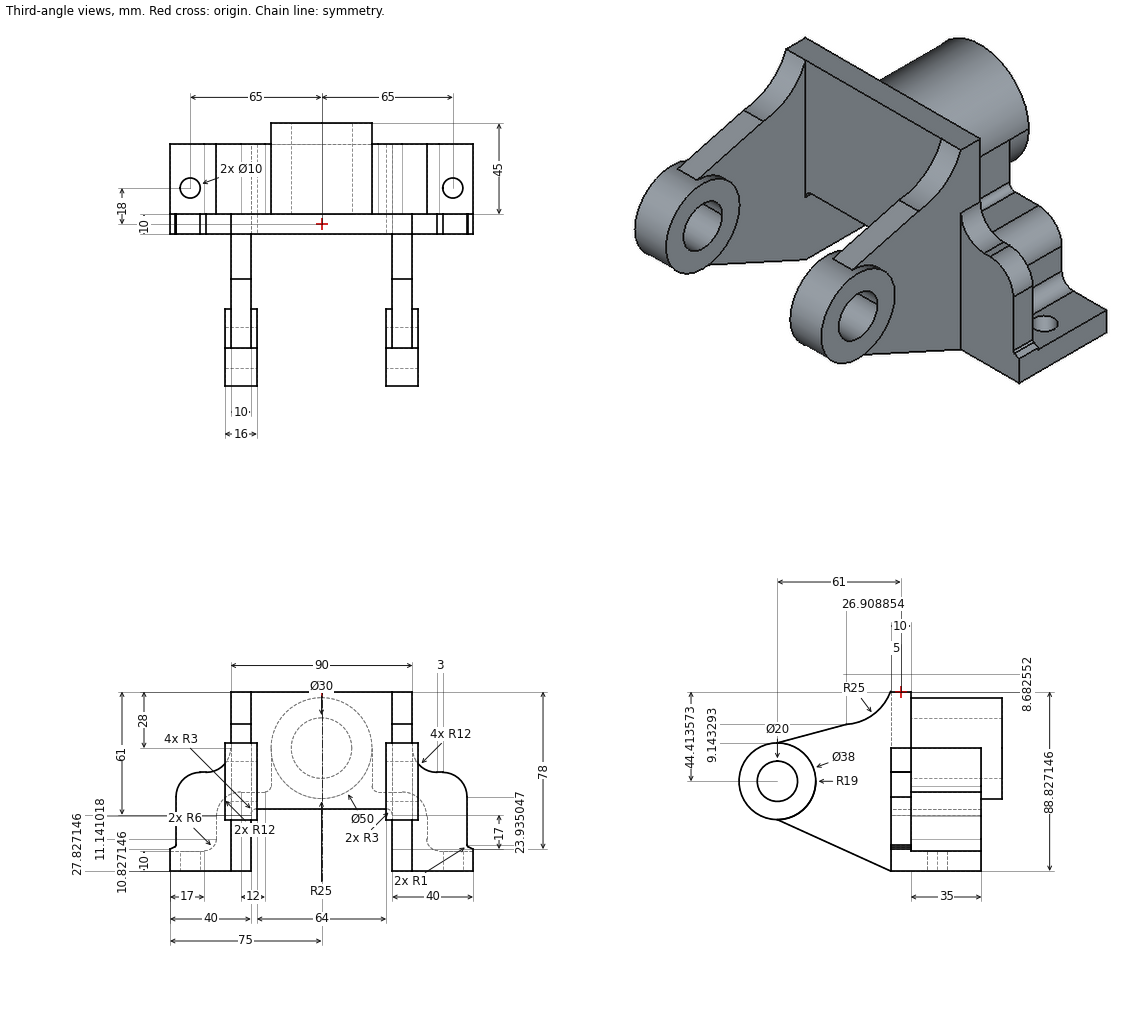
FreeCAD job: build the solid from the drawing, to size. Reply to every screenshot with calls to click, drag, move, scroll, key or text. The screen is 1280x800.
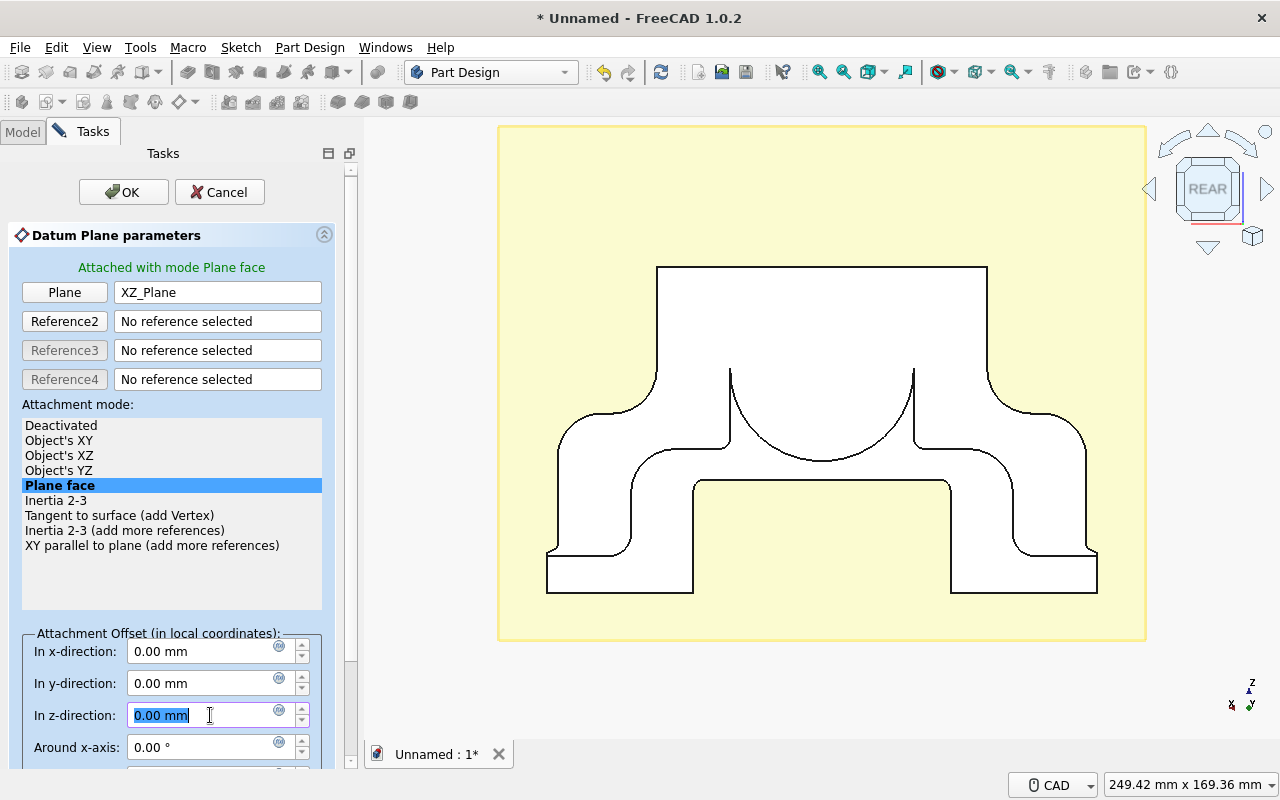
text(-50)
key(Tab)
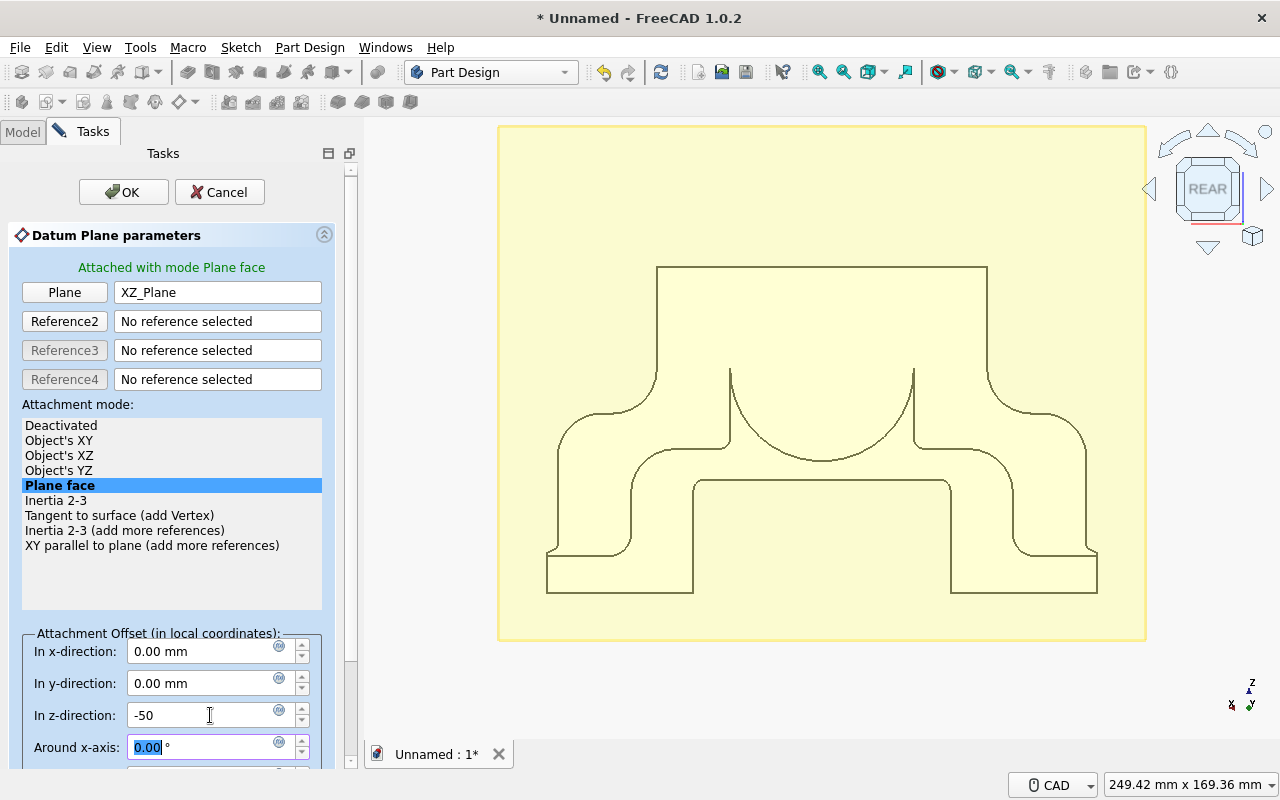
click(124, 192)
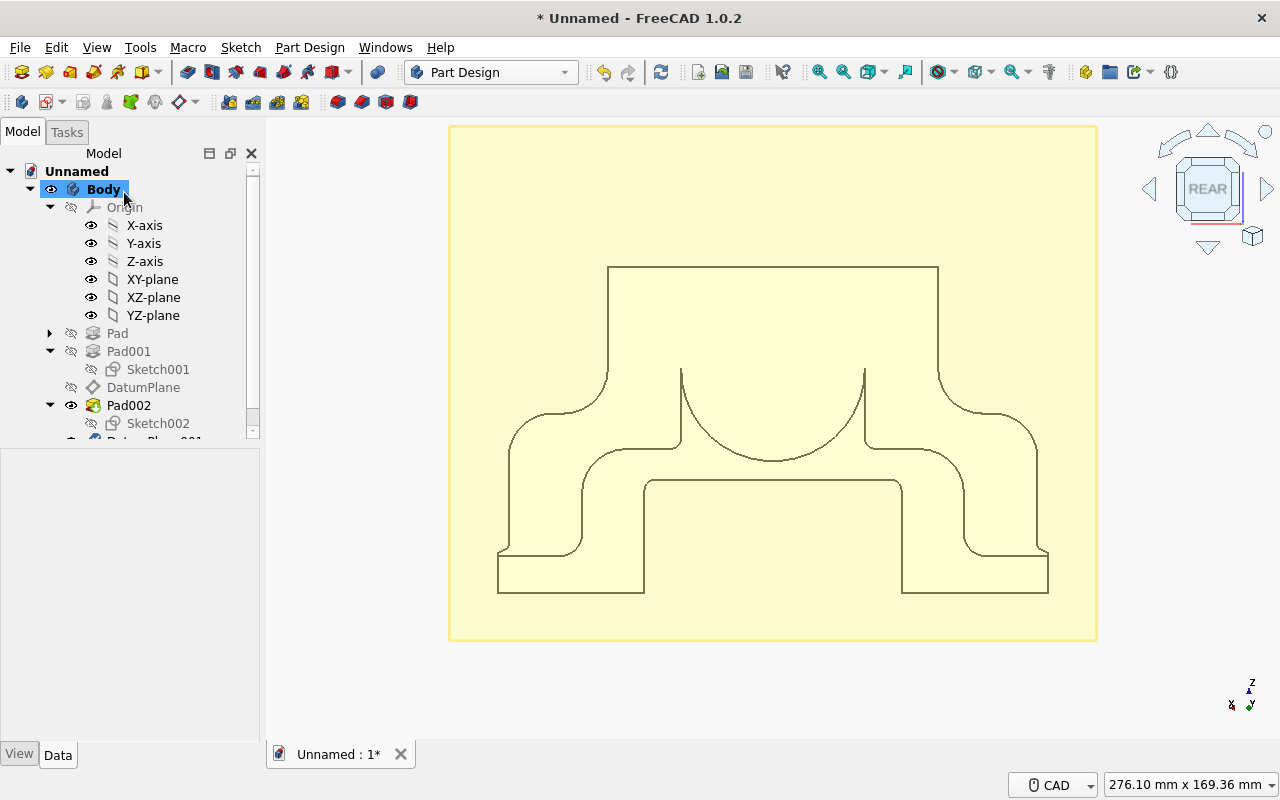
scroll(100, 293, down, 3)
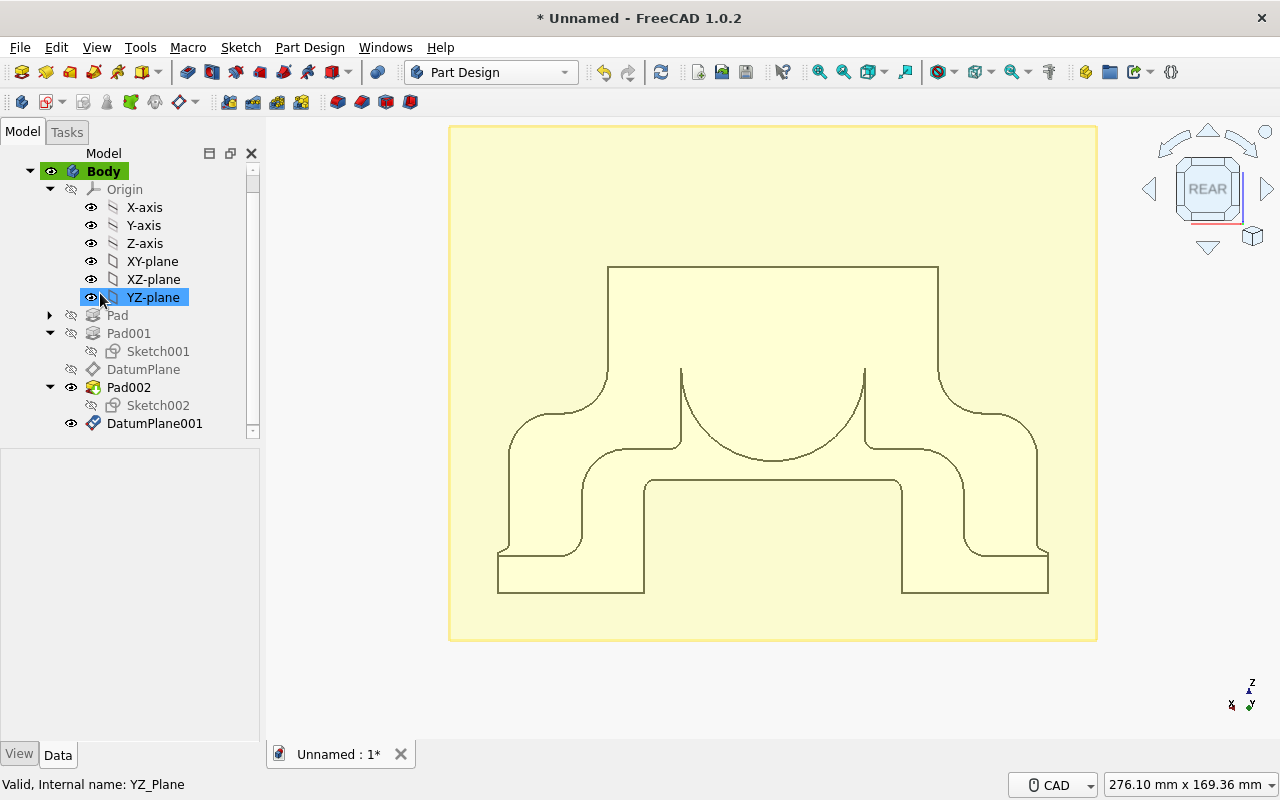
click(116, 423)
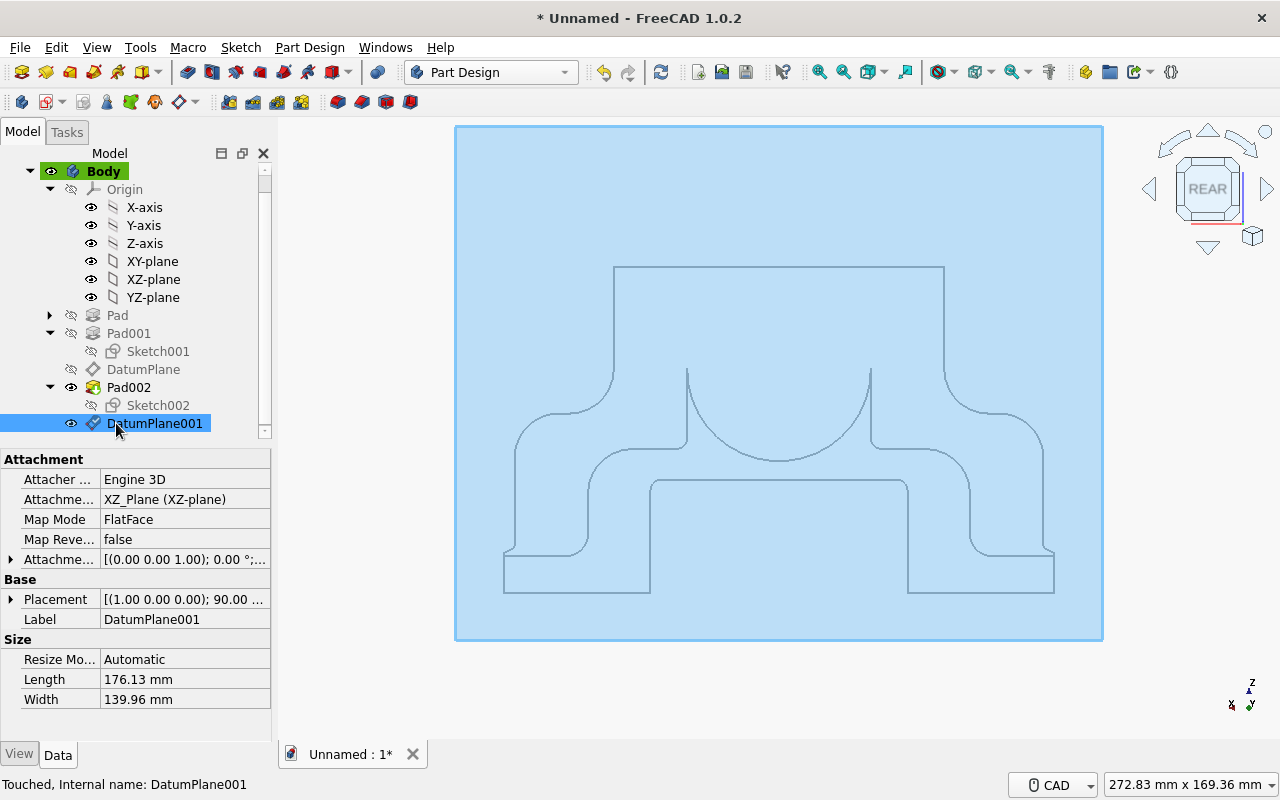
click(46, 102)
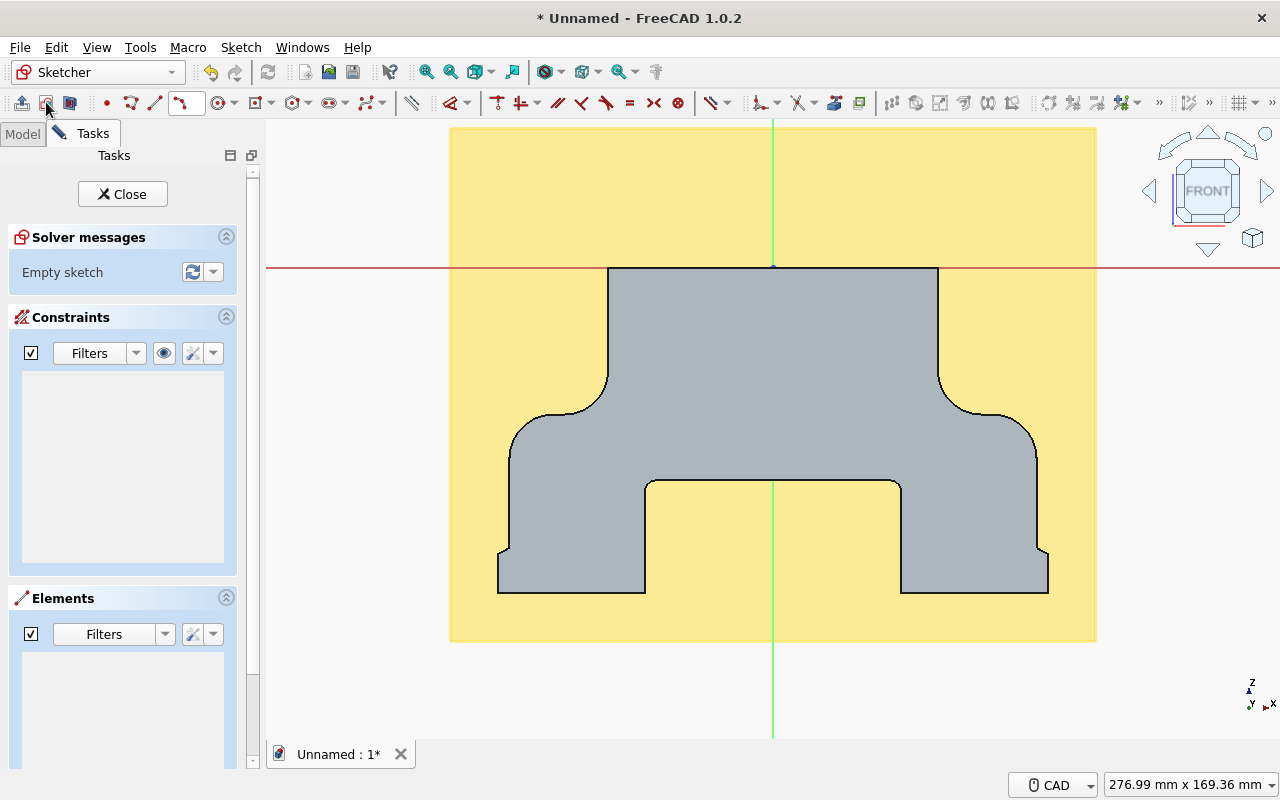
click(70, 104)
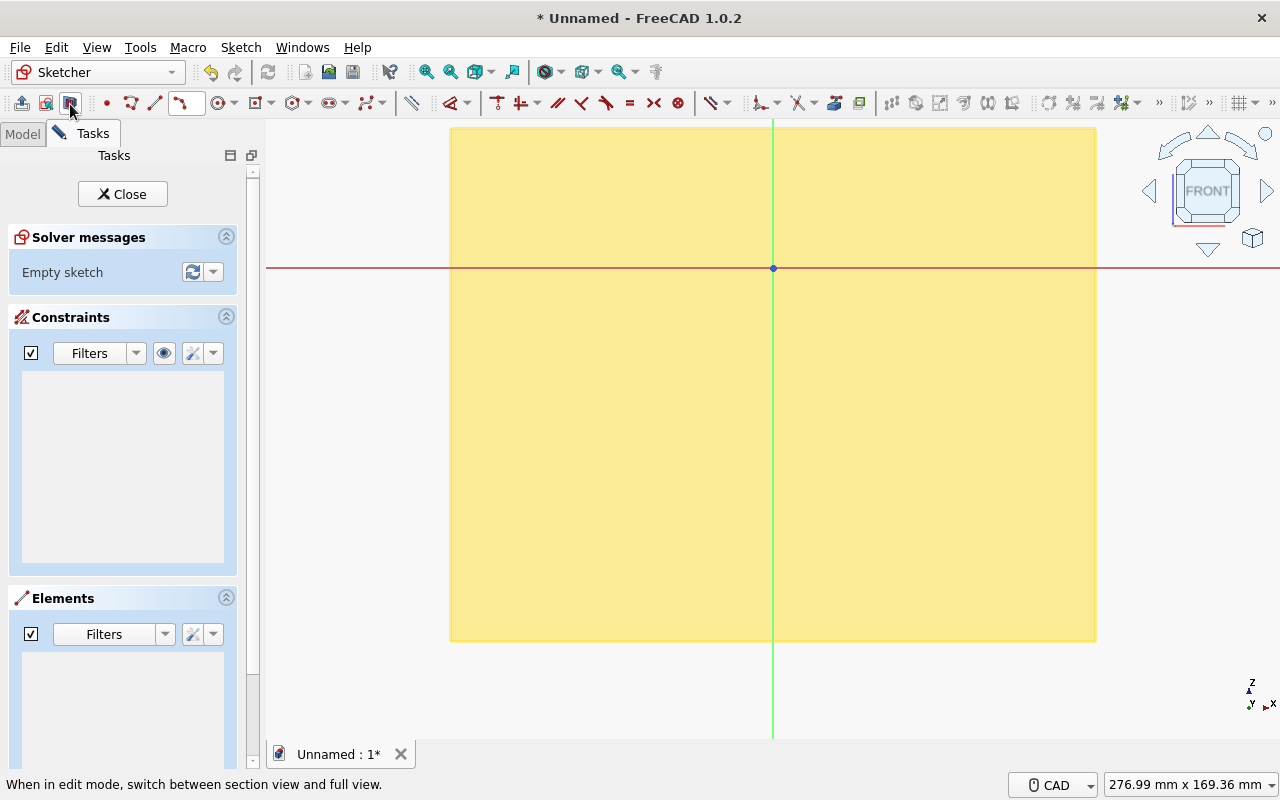
scroll(829, 313, up, 4)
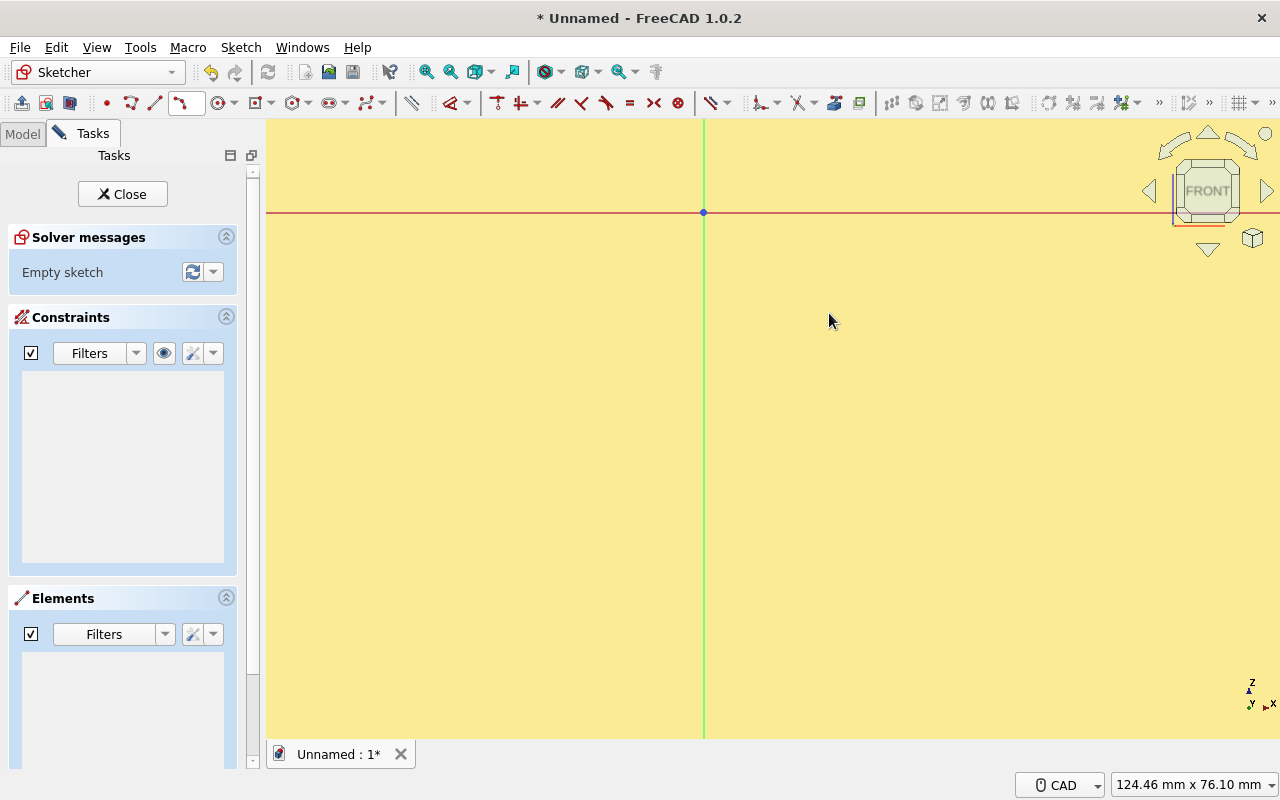
key(g)
key(c)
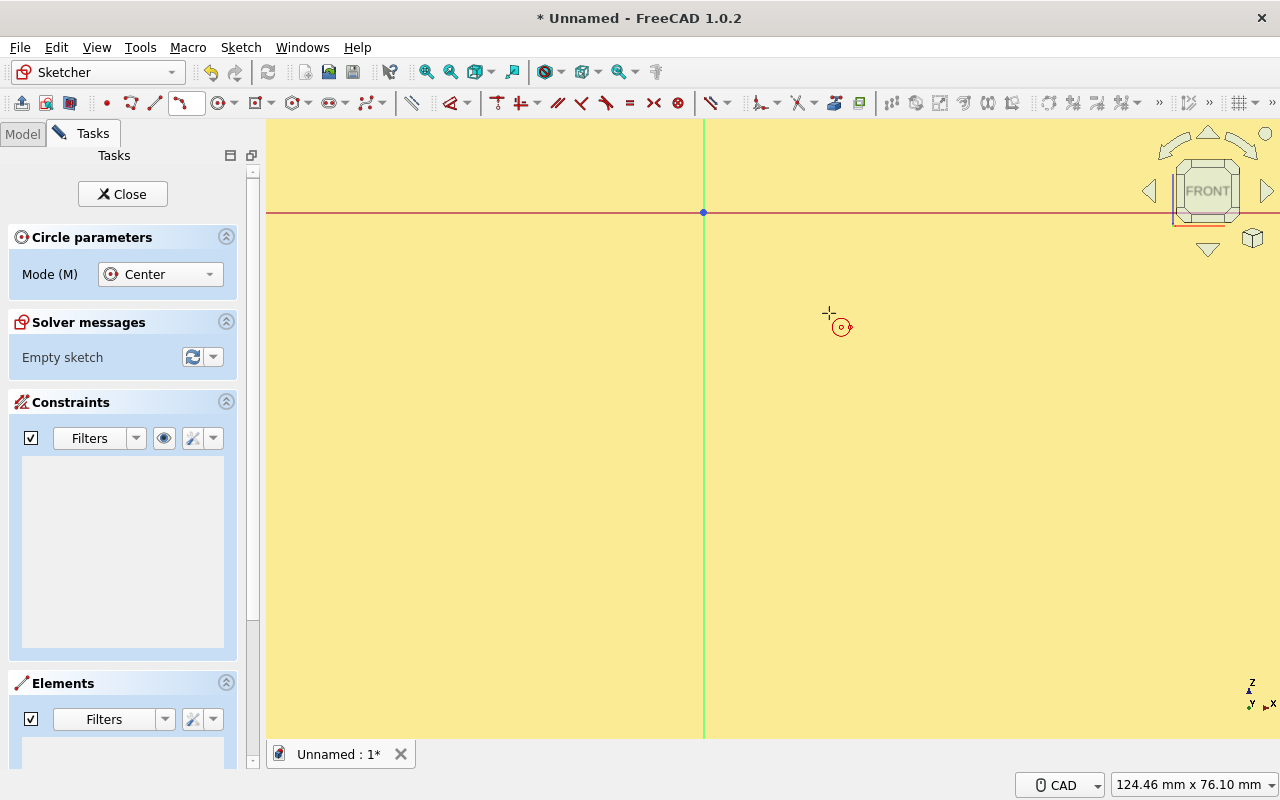
click(704, 441)
click(848, 297)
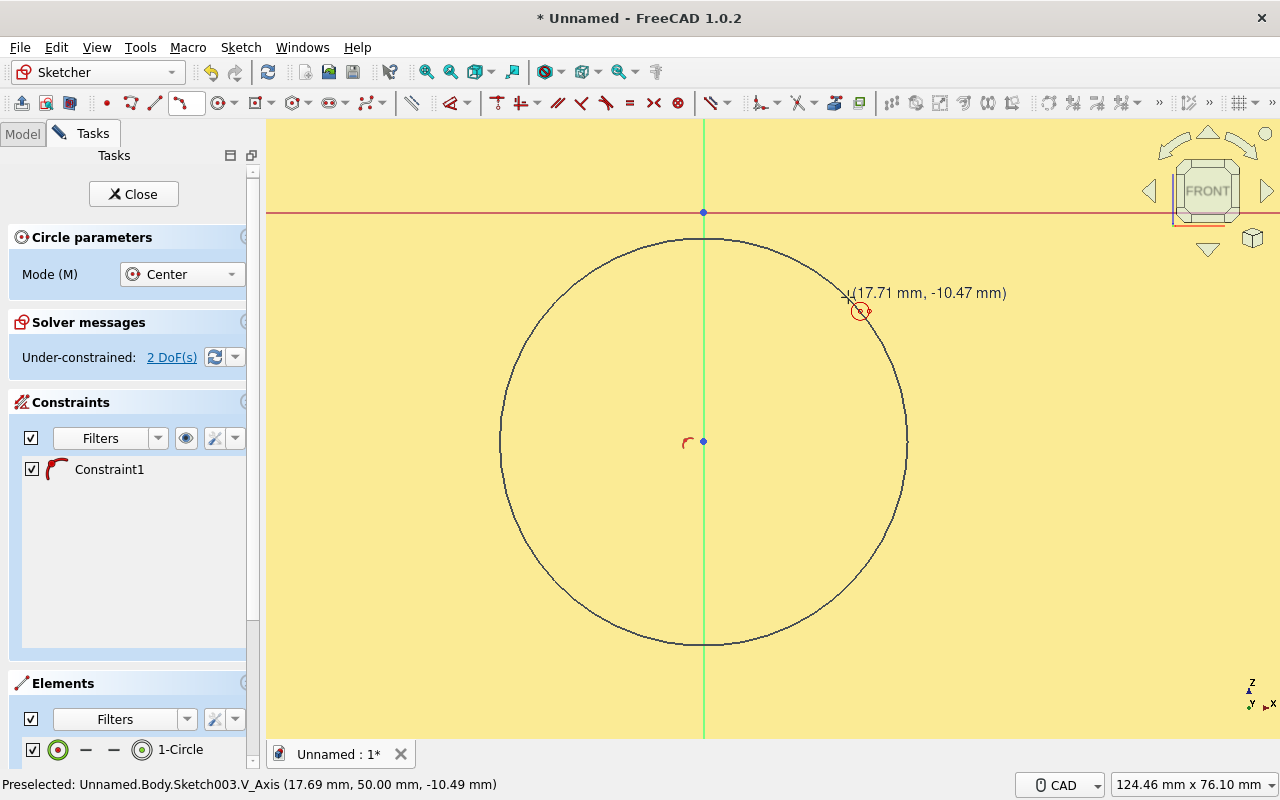
click(704, 442)
click(790, 354)
key(Escape)